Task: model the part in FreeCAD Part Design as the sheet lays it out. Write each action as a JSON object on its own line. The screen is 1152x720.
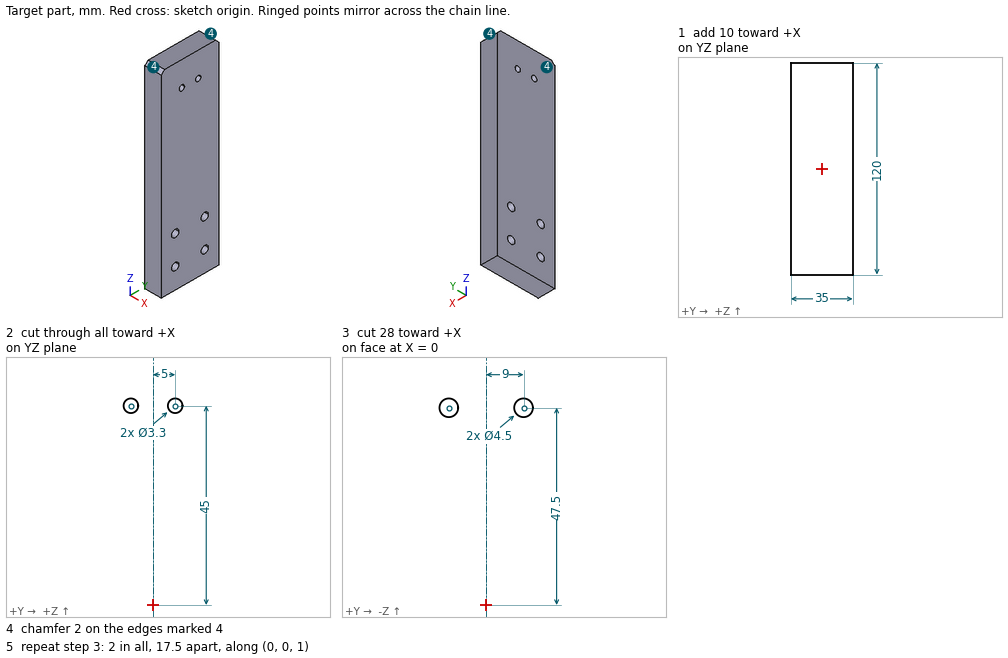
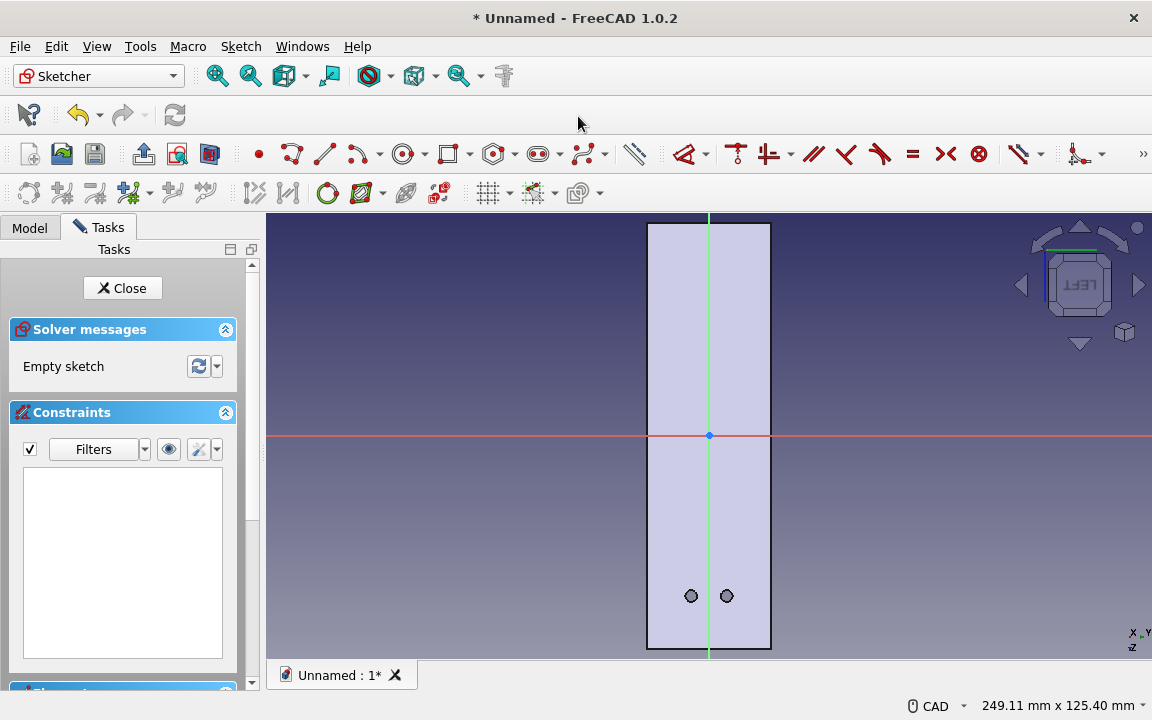
{"action": "scroll", "coordinate": [848, 241], "scroll_direction": "up", "scroll_amount": 2}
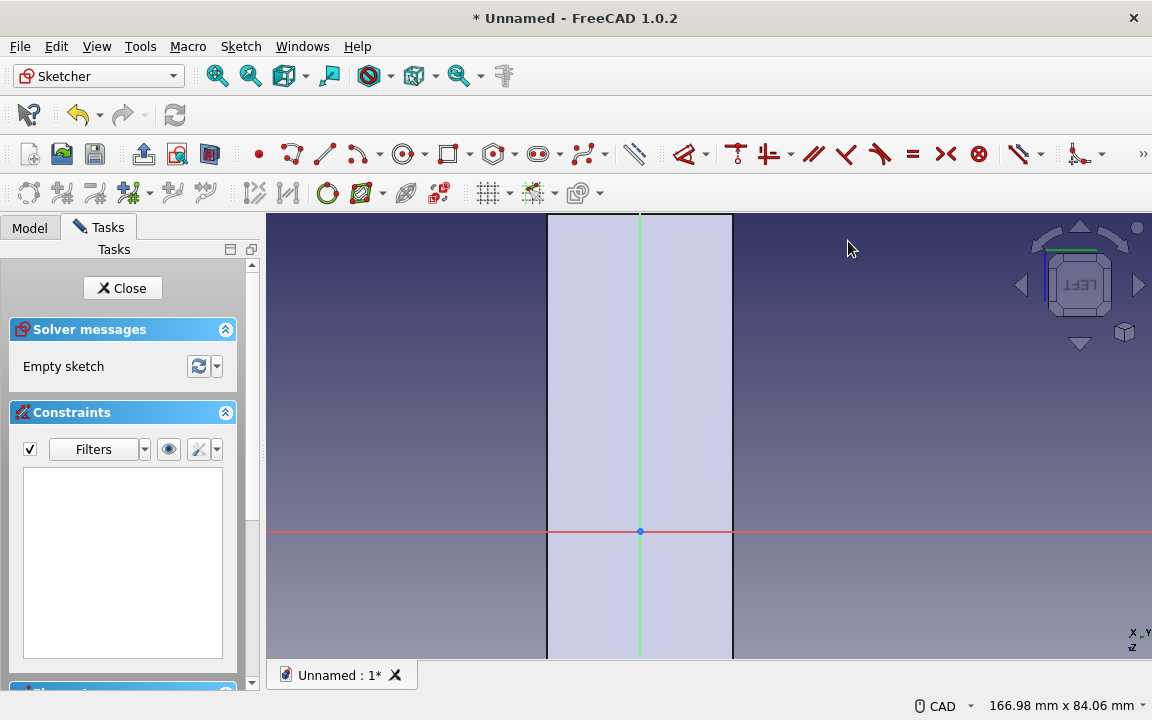
{"action": "left_click", "coordinate": [402, 154]}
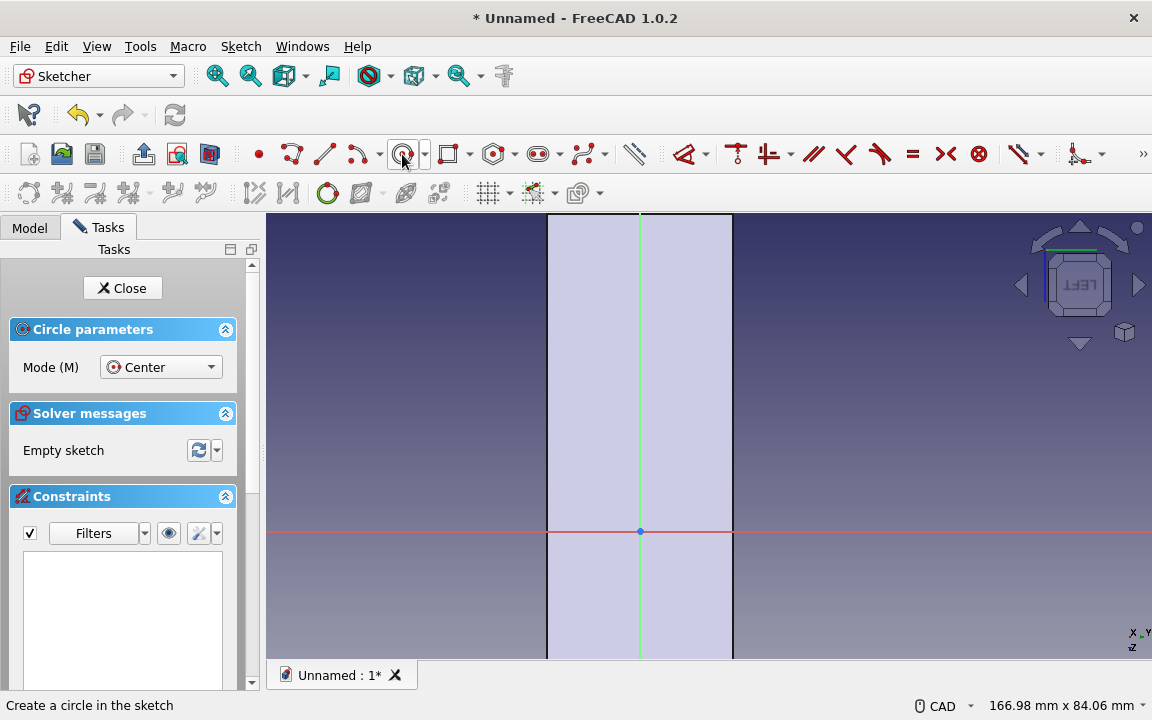
{"action": "scroll", "coordinate": [688, 280], "scroll_direction": "up", "scroll_amount": 4}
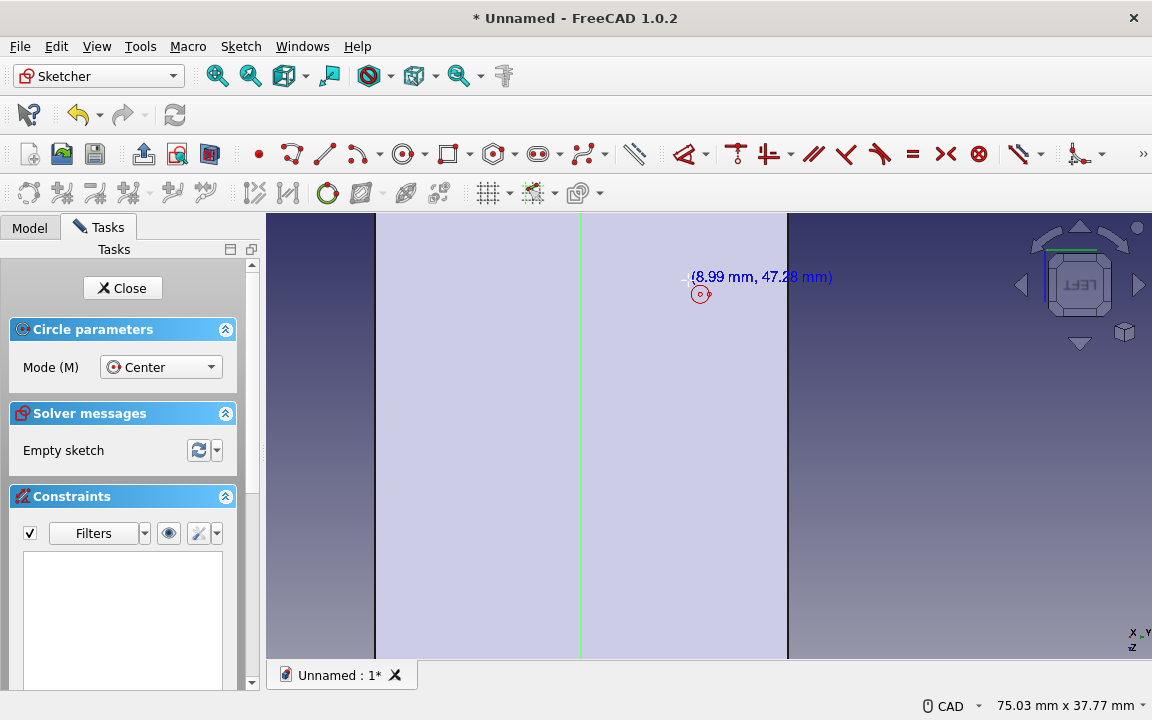
{"action": "left_click", "coordinate": [688, 279]}
{"action": "left_click", "coordinate": [706, 261]}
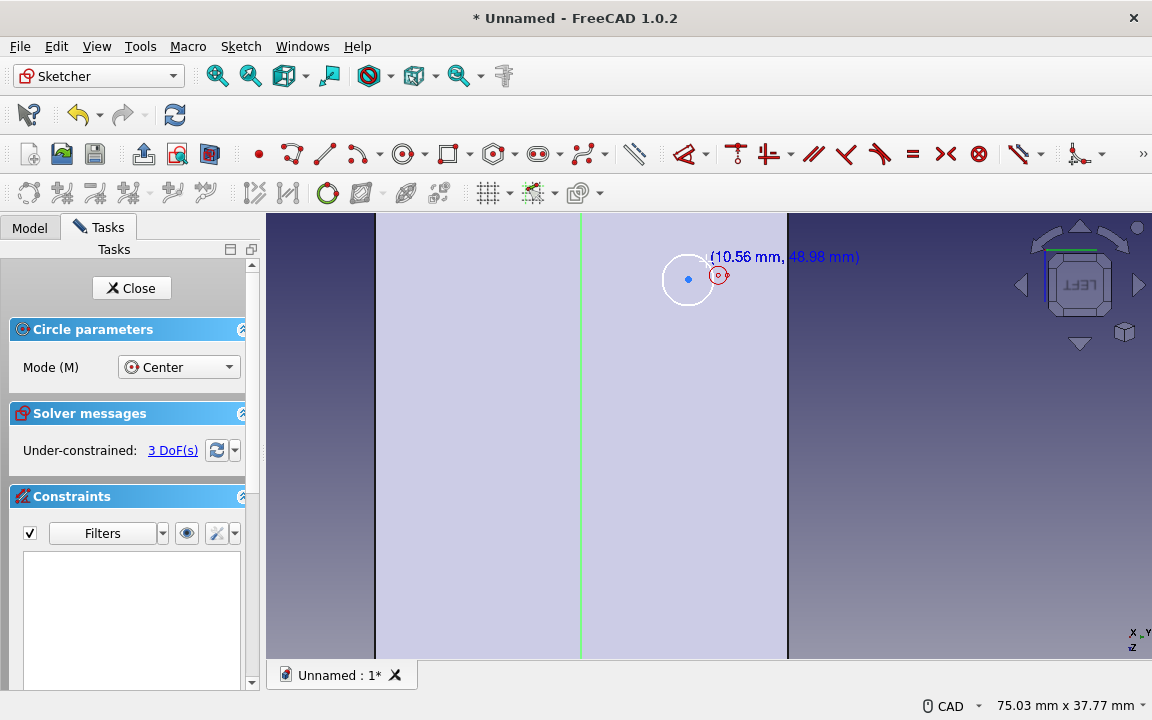
{"action": "left_click", "coordinate": [475, 279]}
{"action": "left_click", "coordinate": [494, 261]}
{"action": "key", "text": "Escape"}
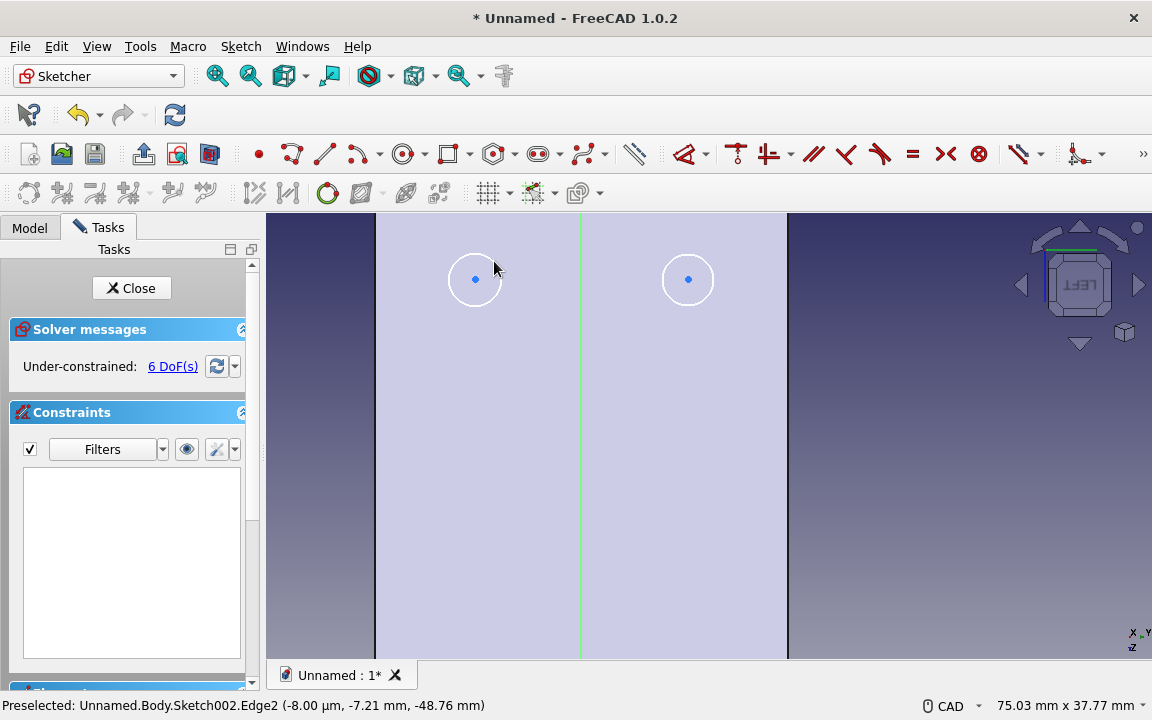
{"action": "left_click", "coordinate": [706, 262]}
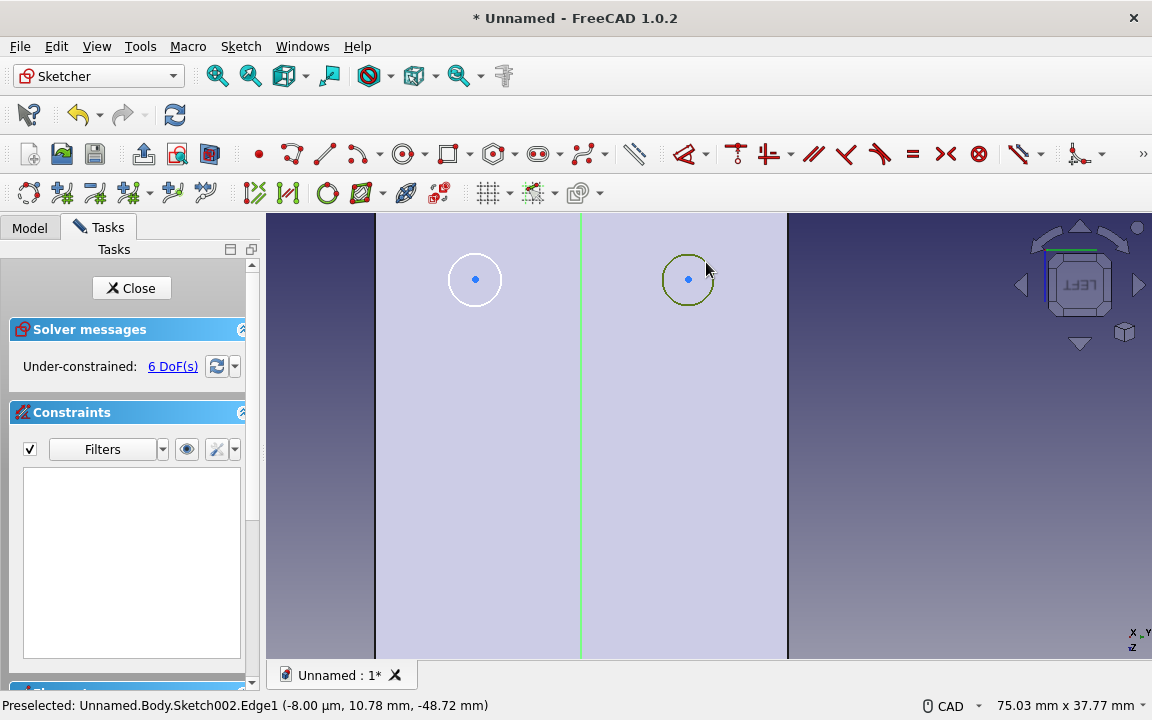
{"action": "left_click", "coordinate": [493, 261]}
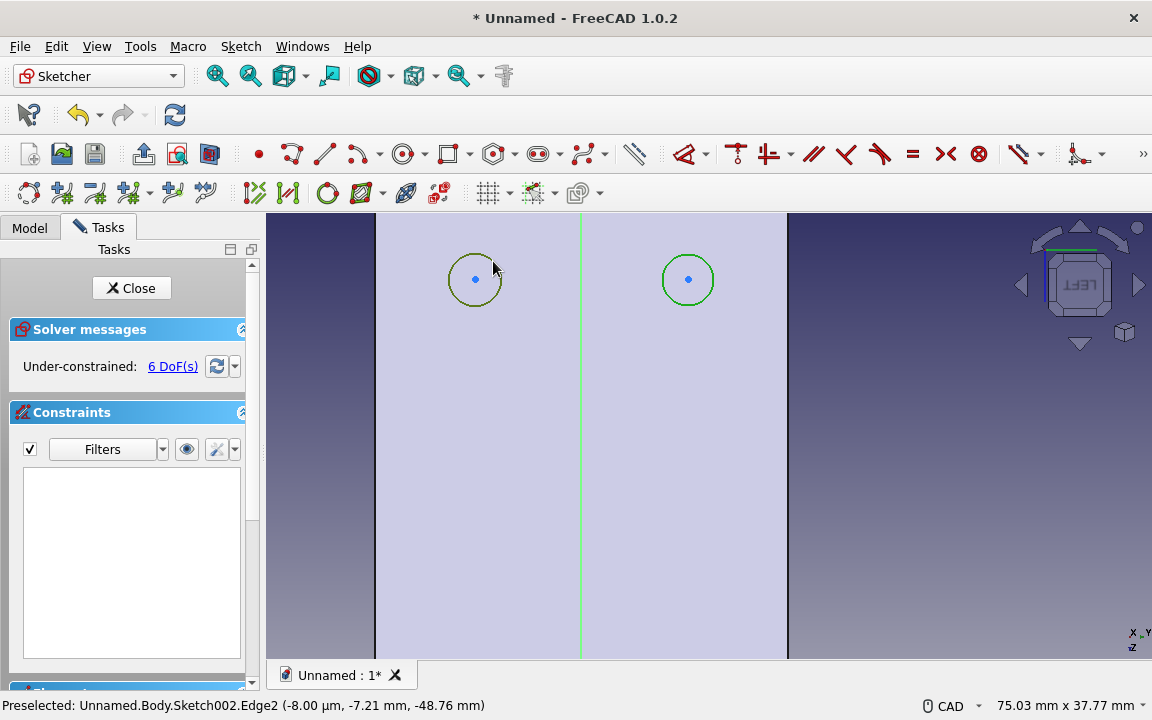
{"action": "left_click", "coordinate": [913, 154]}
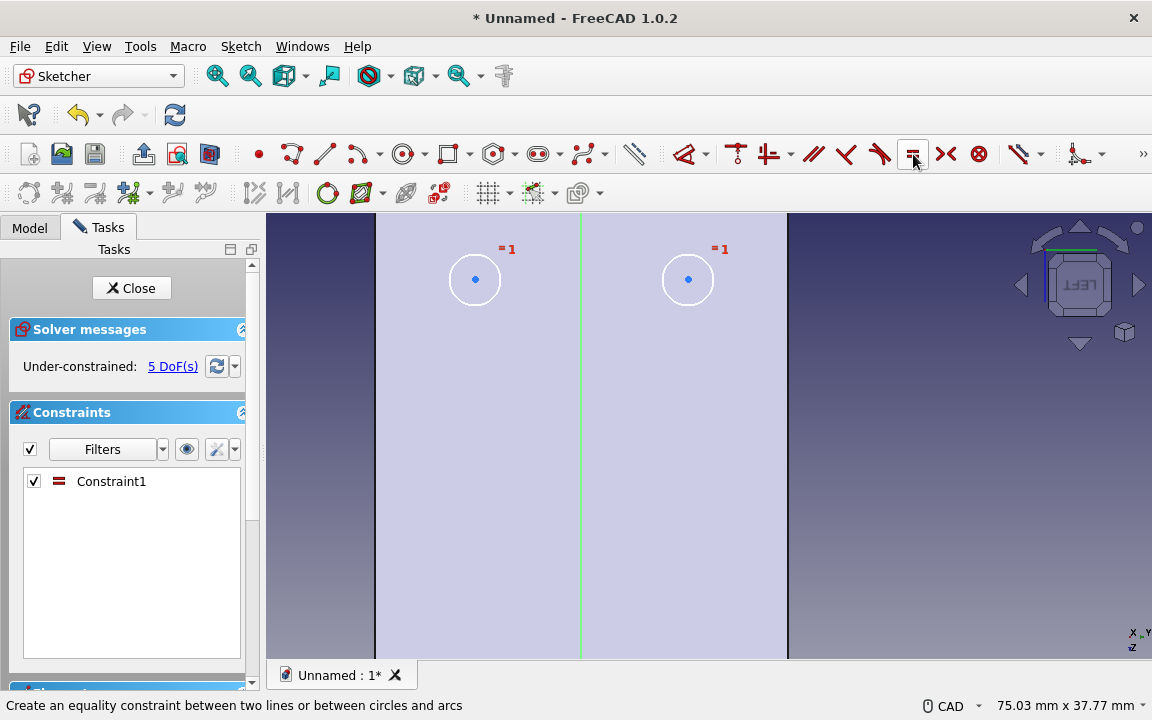
{"action": "left_click", "coordinate": [688, 280]}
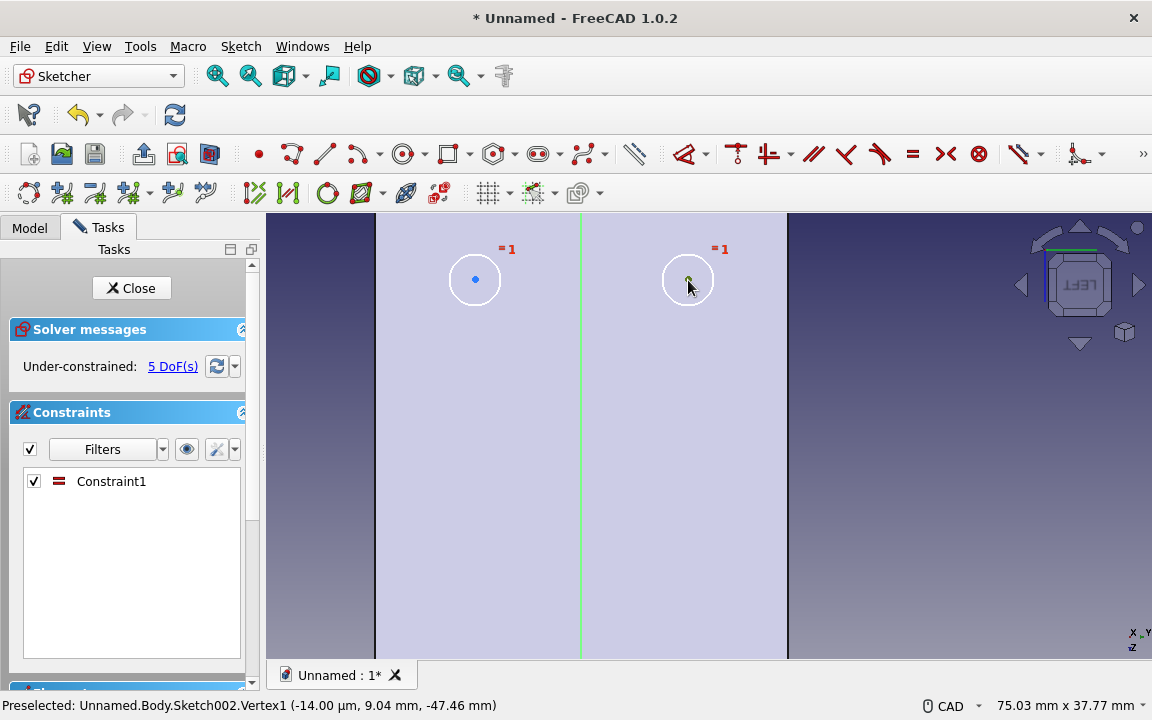
{"action": "left_click", "coordinate": [475, 280]}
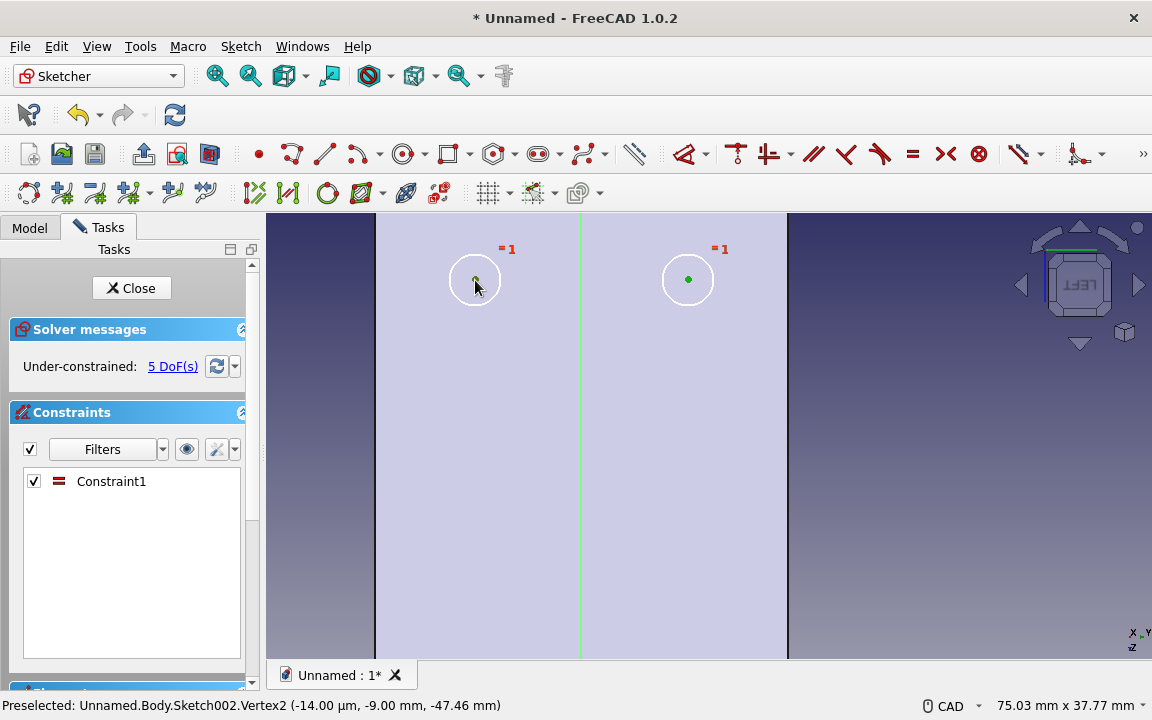
{"action": "left_click", "coordinate": [581, 603]}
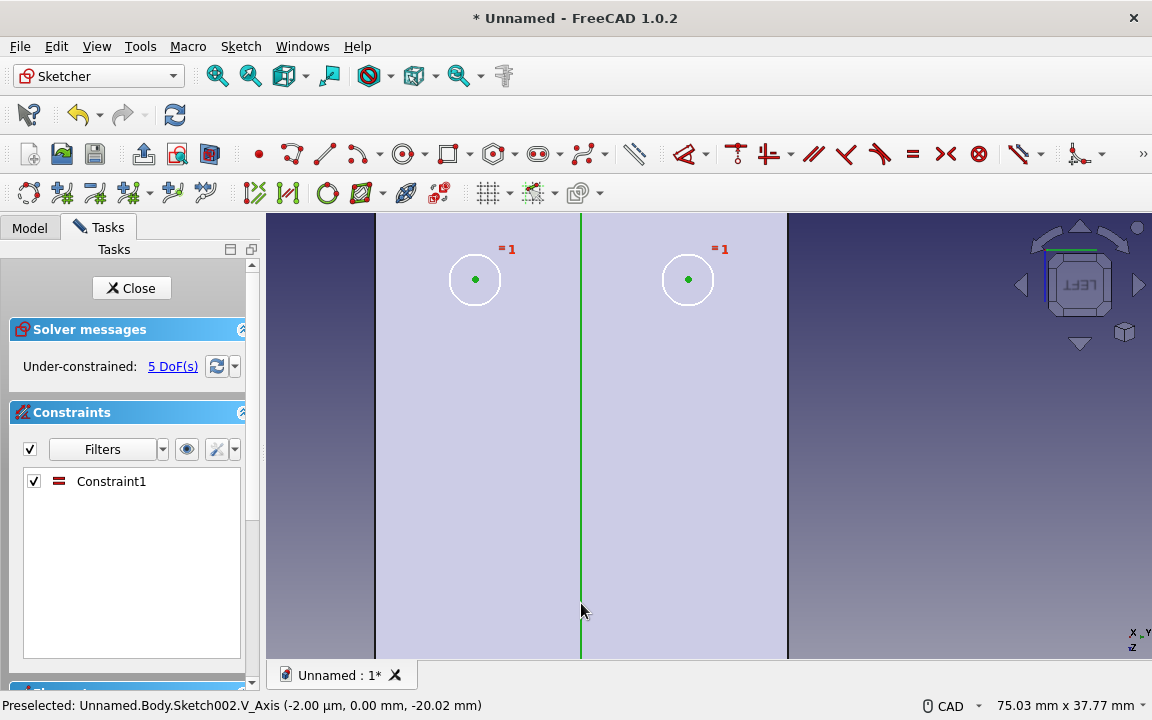
{"action": "left_click", "coordinate": [946, 154]}